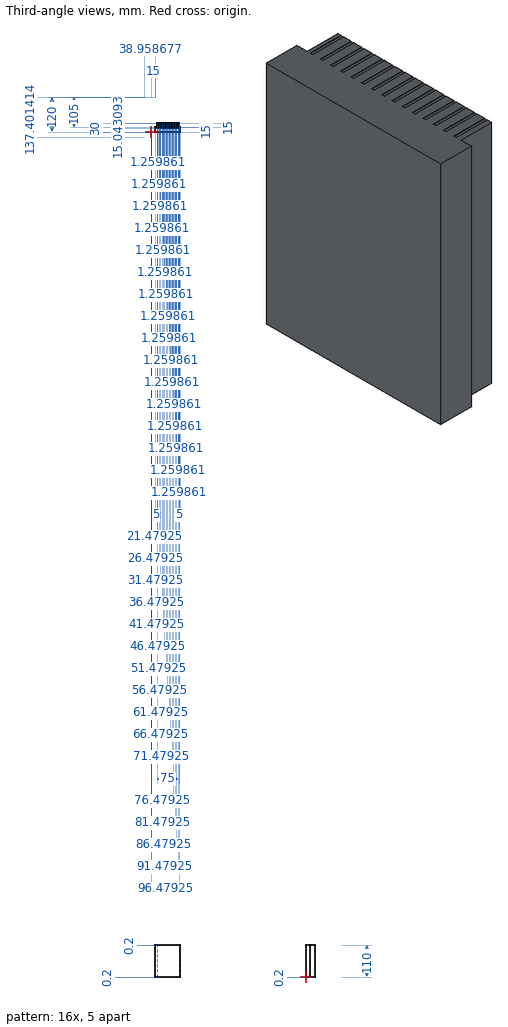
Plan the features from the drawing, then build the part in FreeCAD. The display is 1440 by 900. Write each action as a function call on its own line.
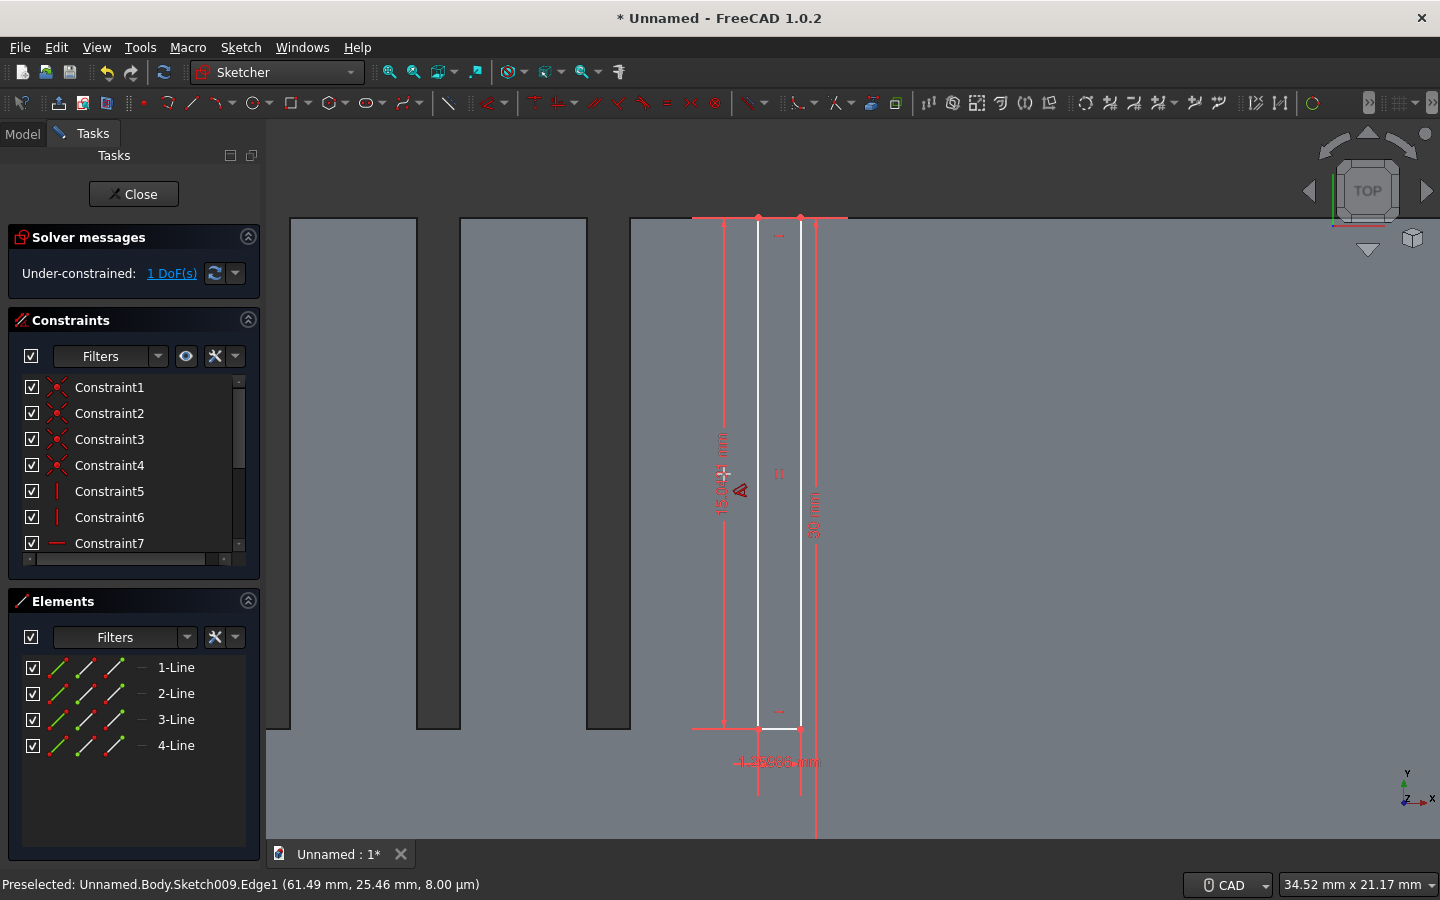
click(758, 218)
click(526, 184)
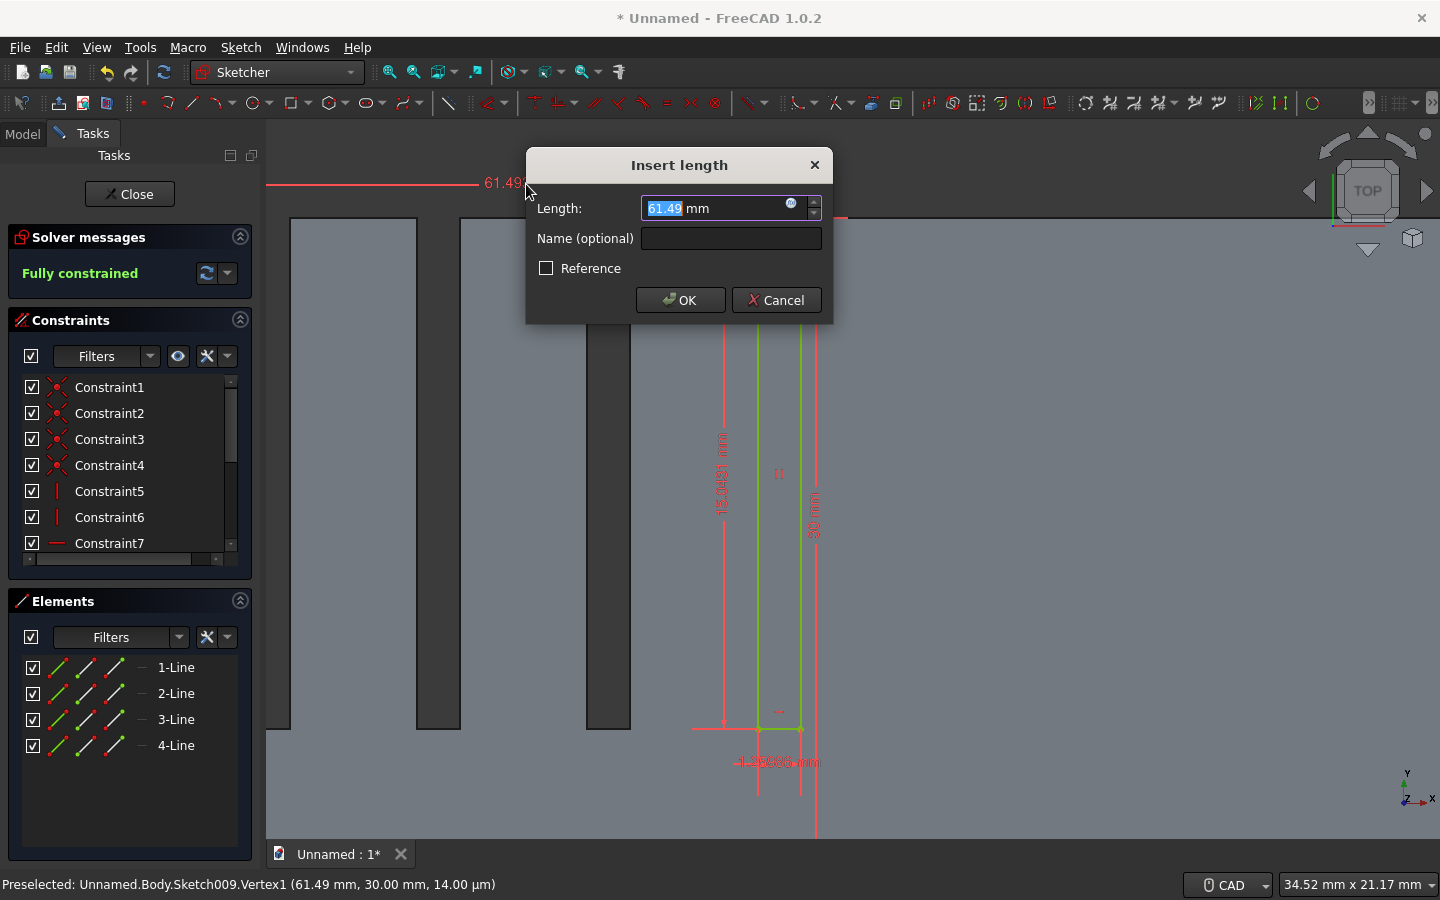
text(61.47925)
key(Return)
key(Escape)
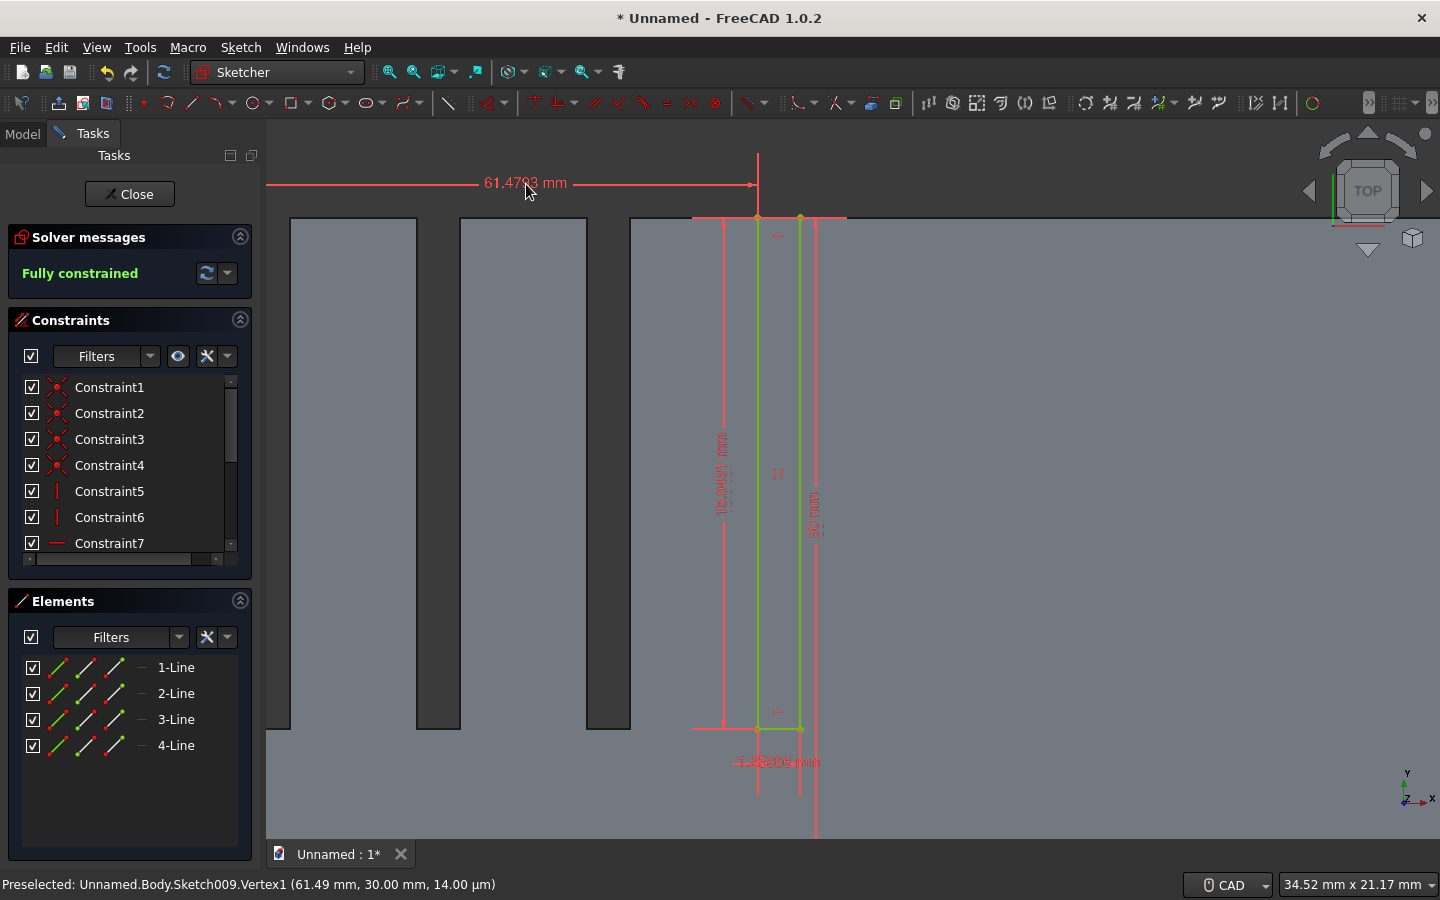
click(130, 194)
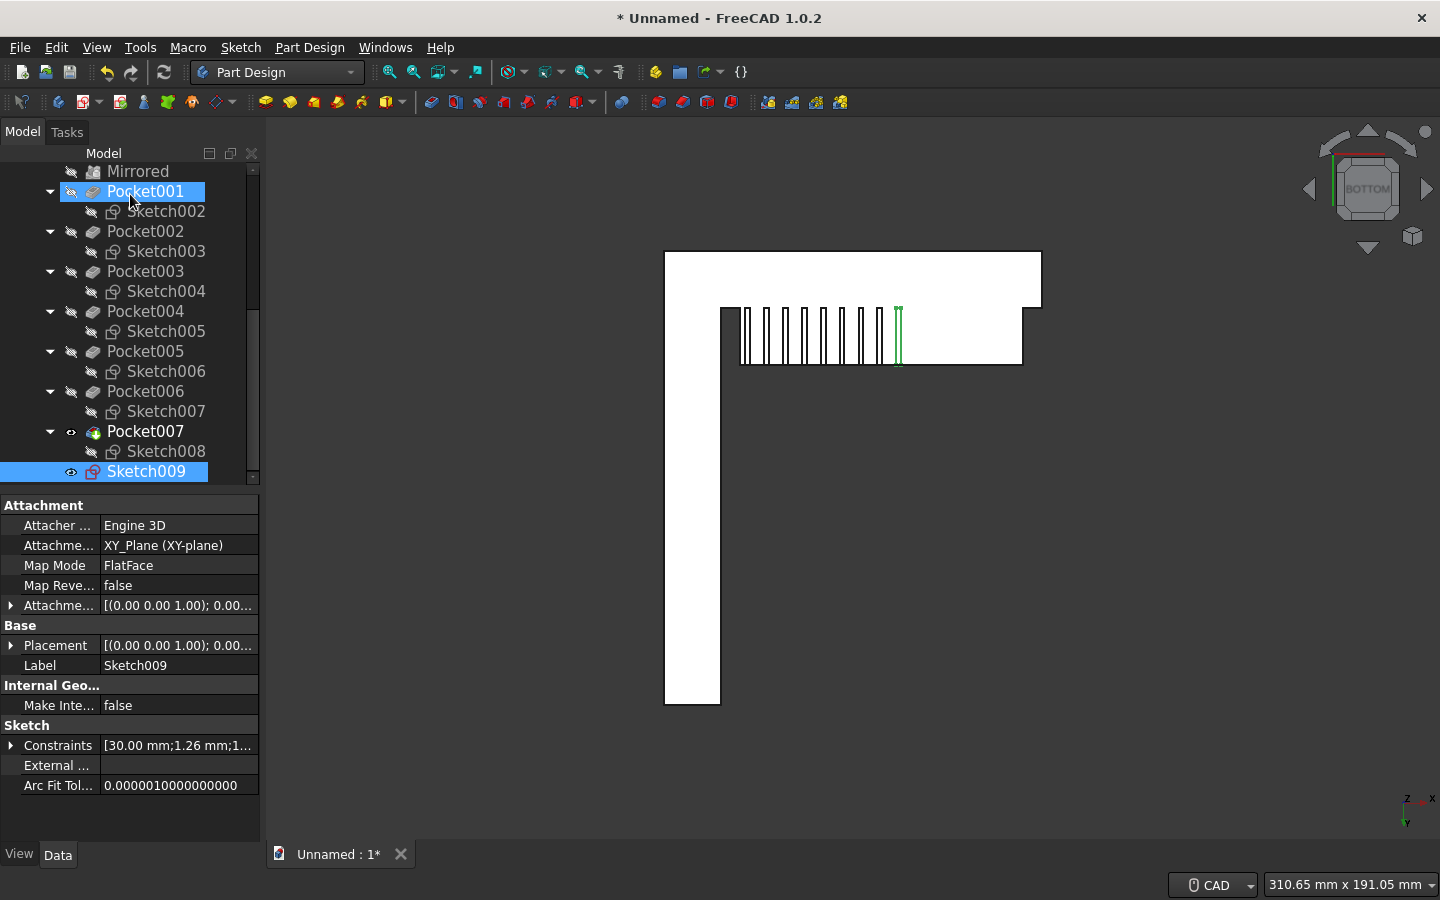
click(432, 102)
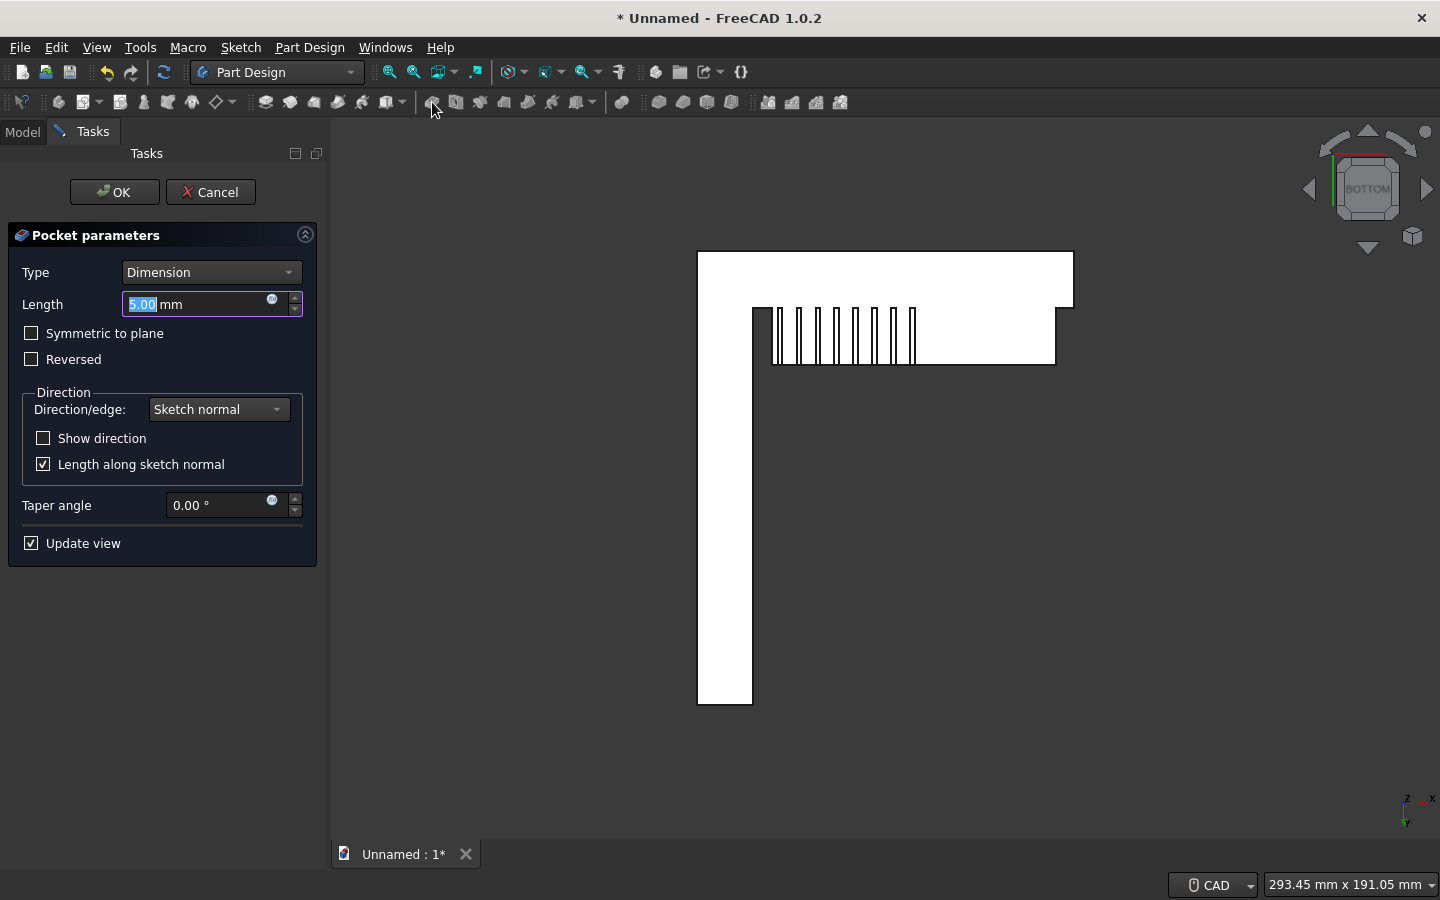
text(0.2)
key(Tab)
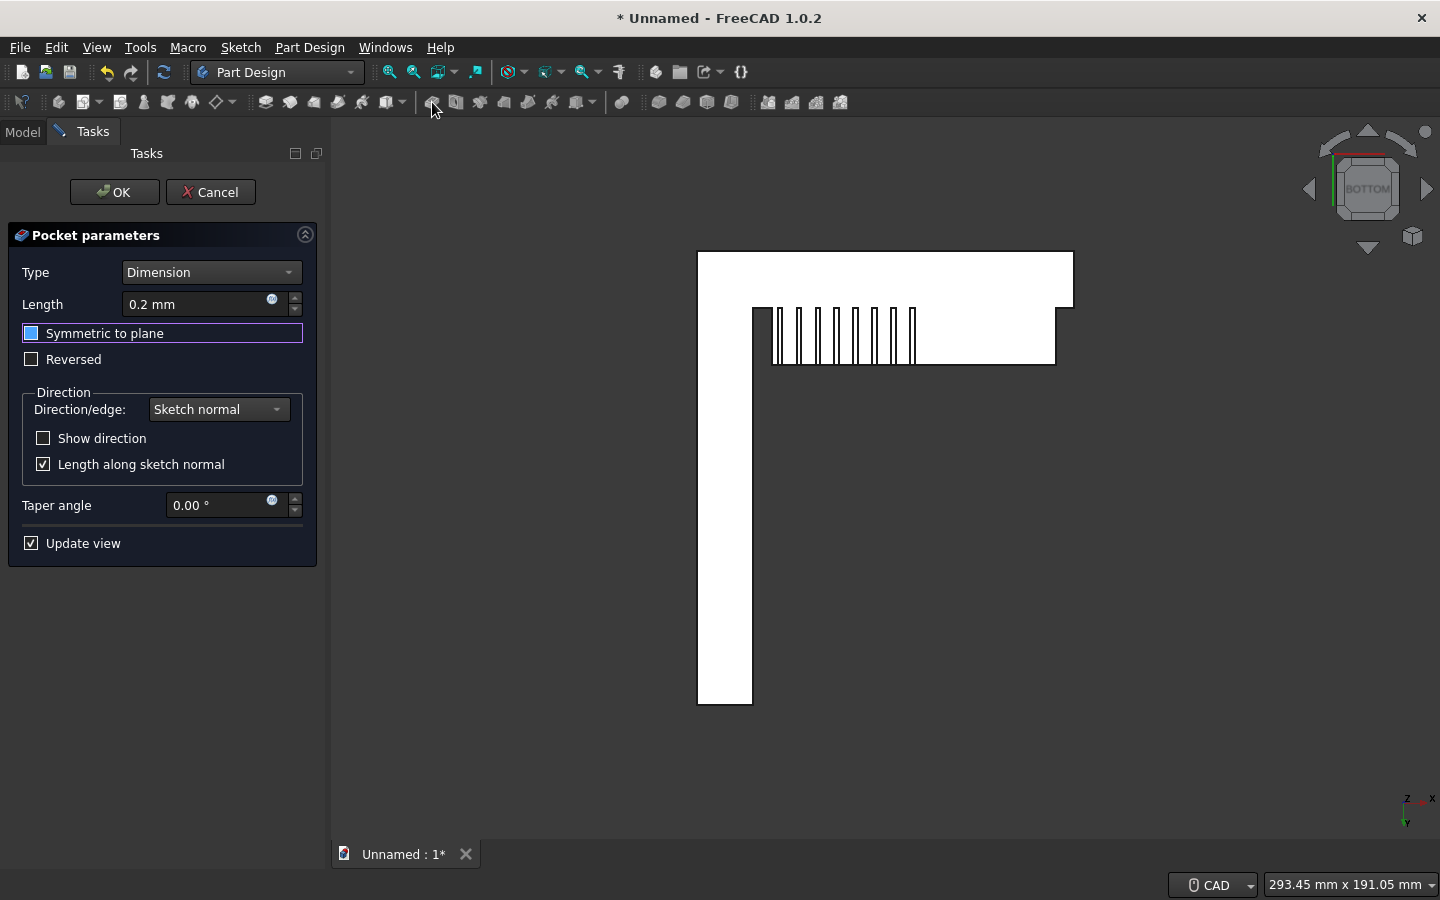
click(30, 359)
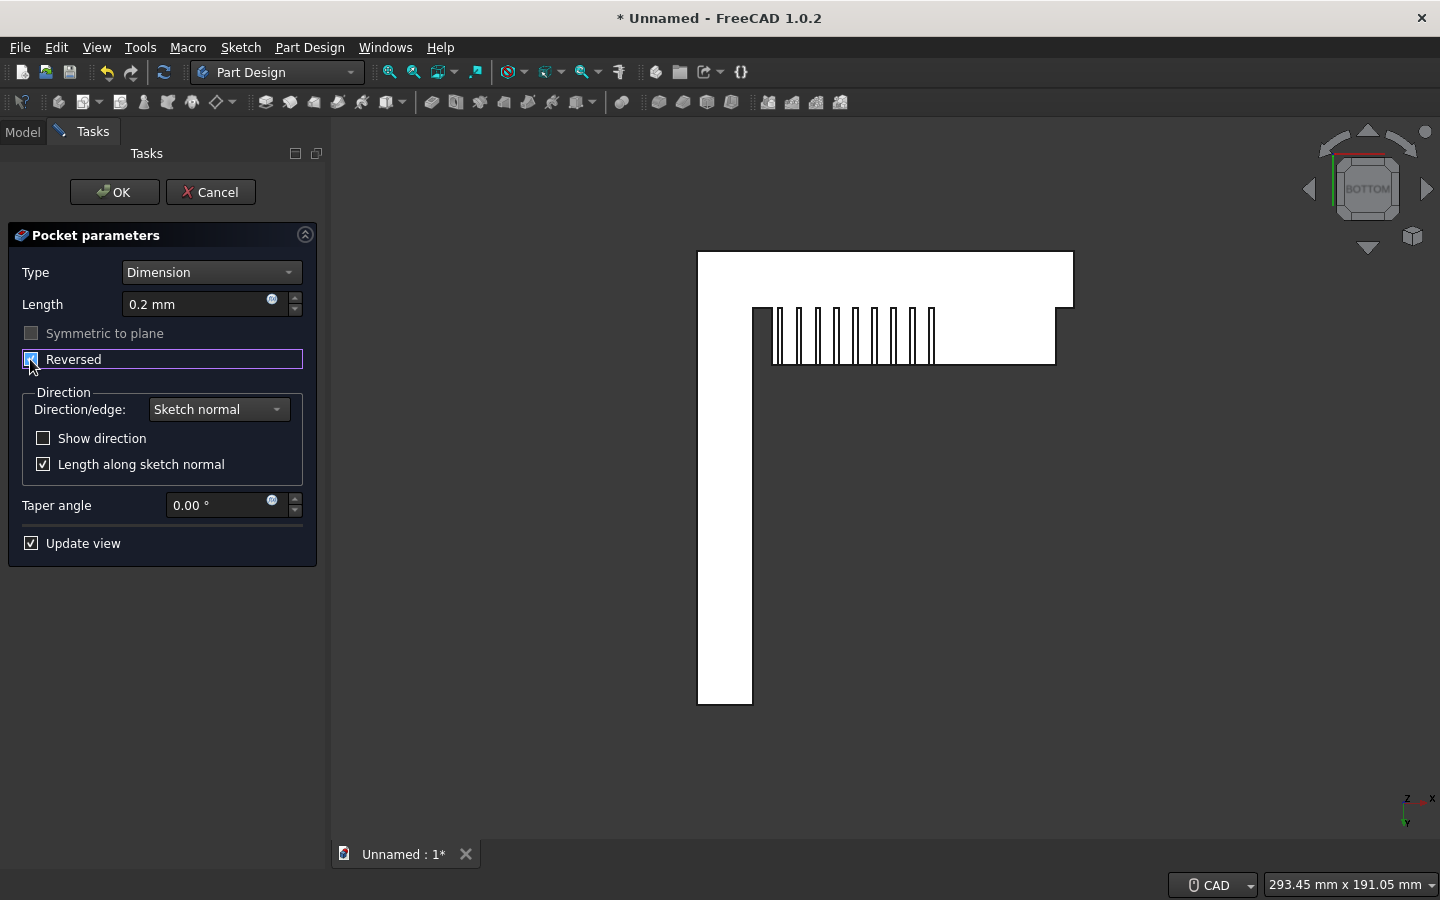
click(115, 192)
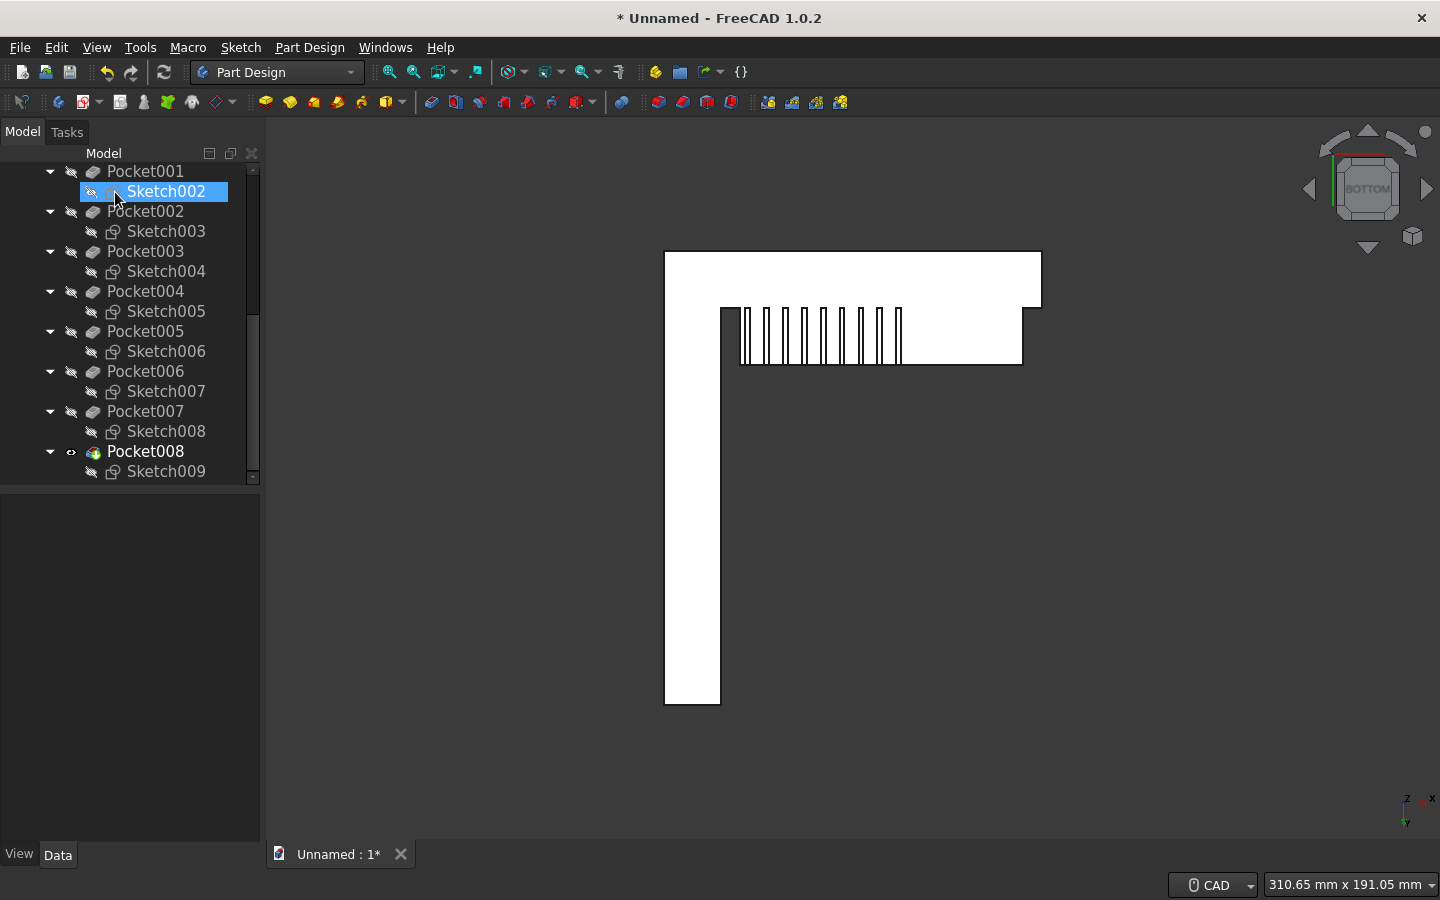
click(84, 102)